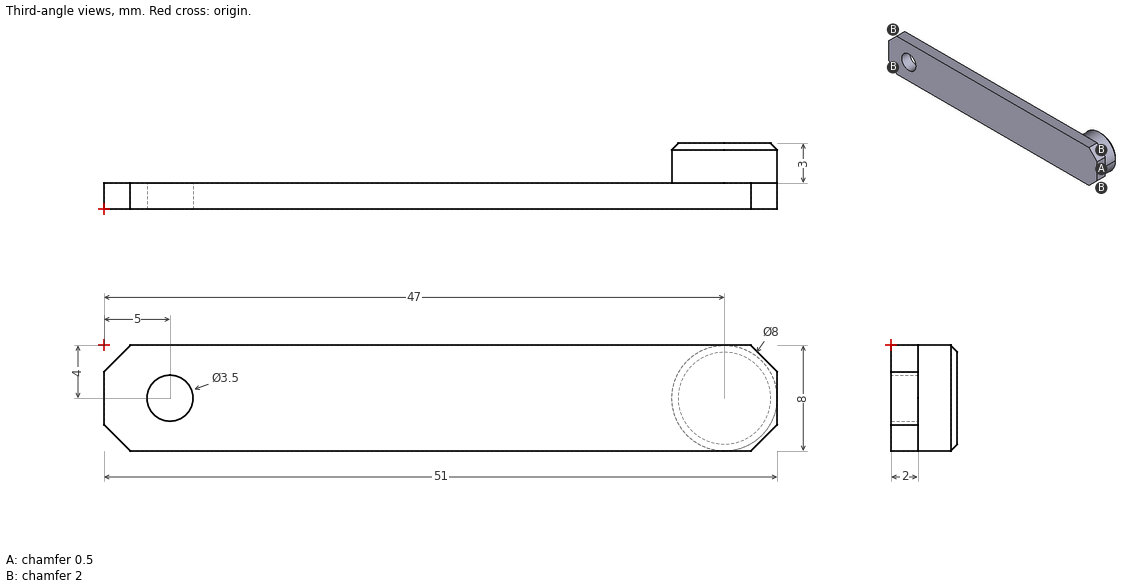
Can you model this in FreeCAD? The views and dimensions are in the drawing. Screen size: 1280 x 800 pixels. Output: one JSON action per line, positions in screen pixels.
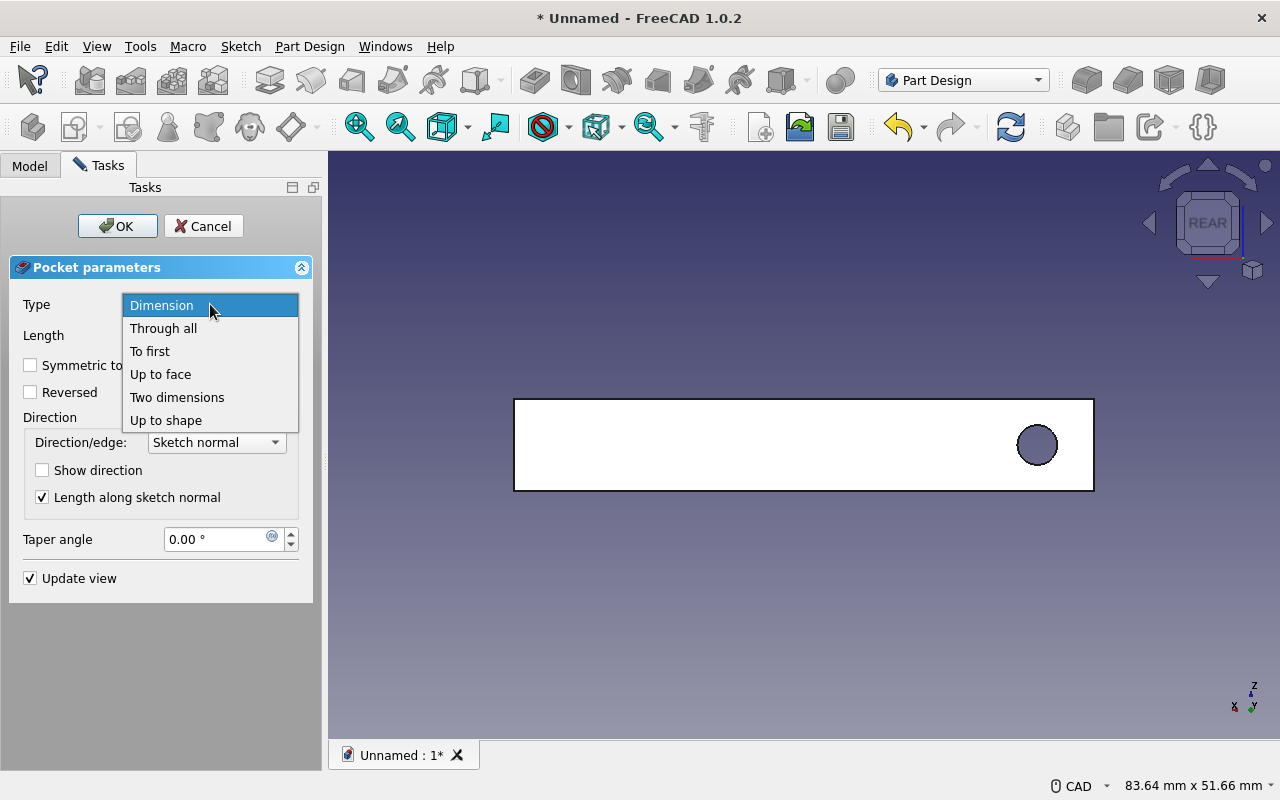
{"action": "left_click", "coordinate": [208, 328]}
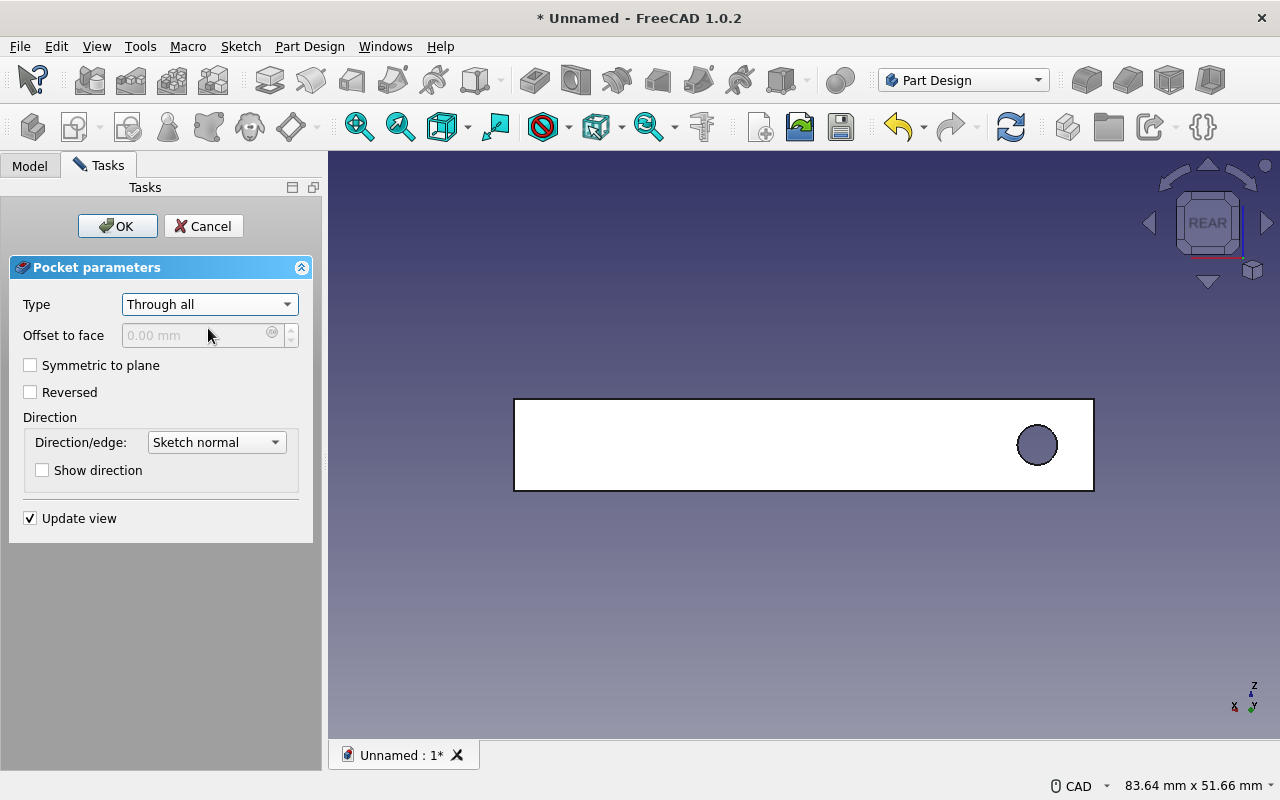
{"action": "left_click", "coordinate": [118, 226]}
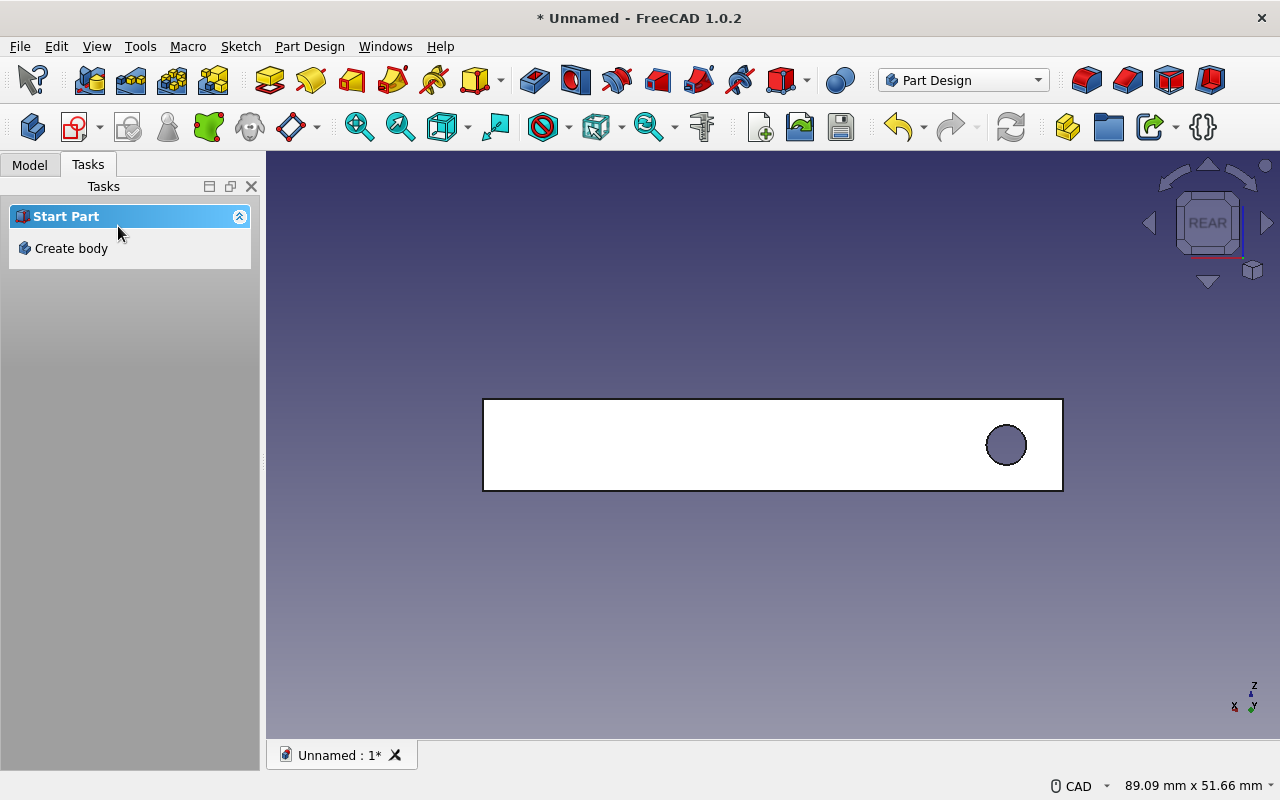
{"action": "left_click", "coordinate": [607, 444]}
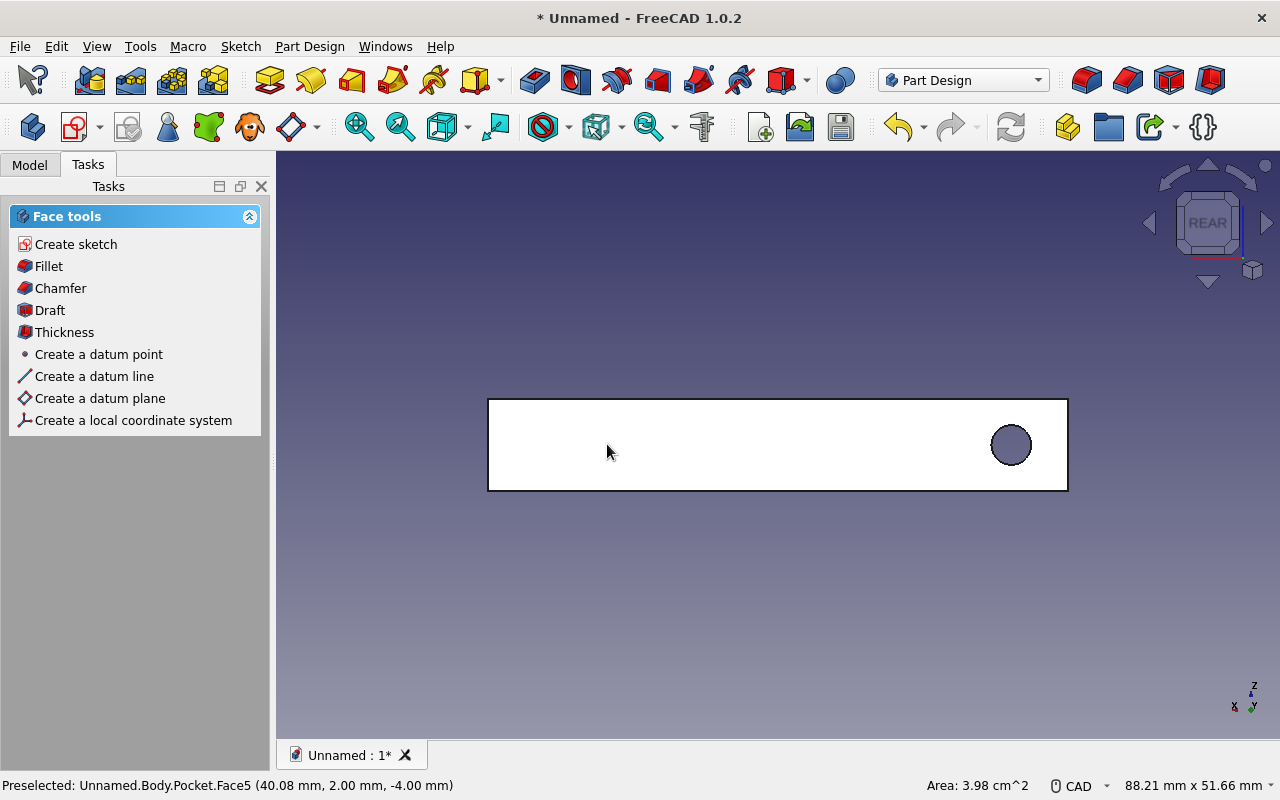
{"action": "left_click", "coordinate": [74, 128]}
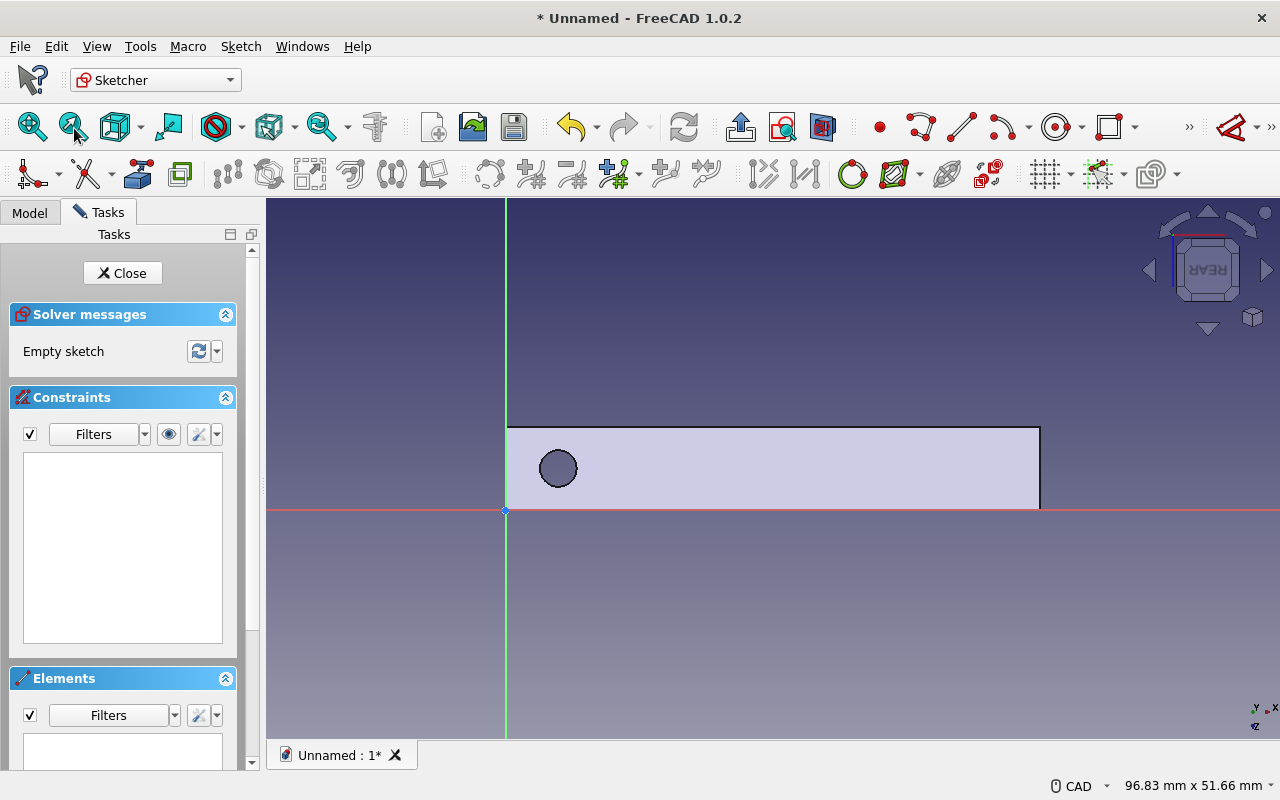
{"action": "scroll", "coordinate": [1094, 468], "scroll_direction": "up", "scroll_amount": 7}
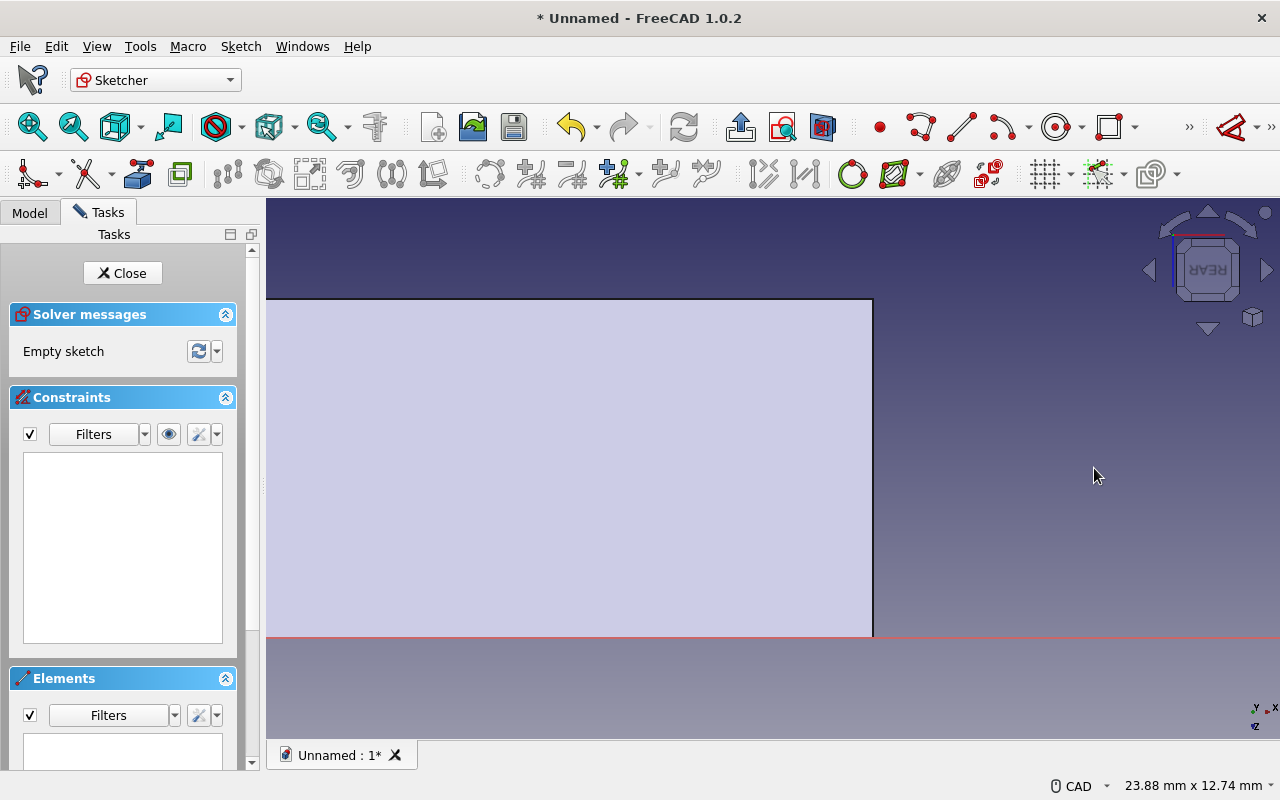
{"action": "key", "text": "g c"}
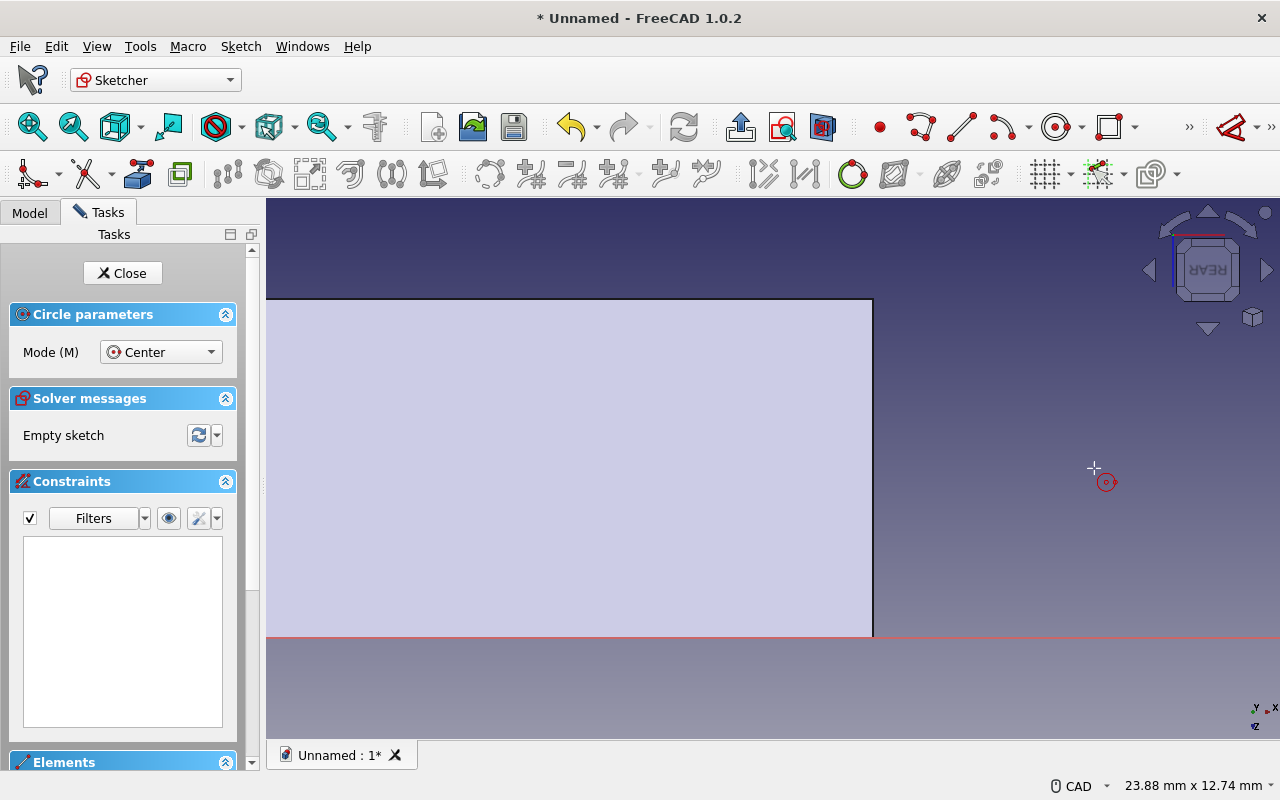
{"action": "left_click", "coordinate": [703, 468]}
{"action": "mouse_move", "coordinate": [823, 348]}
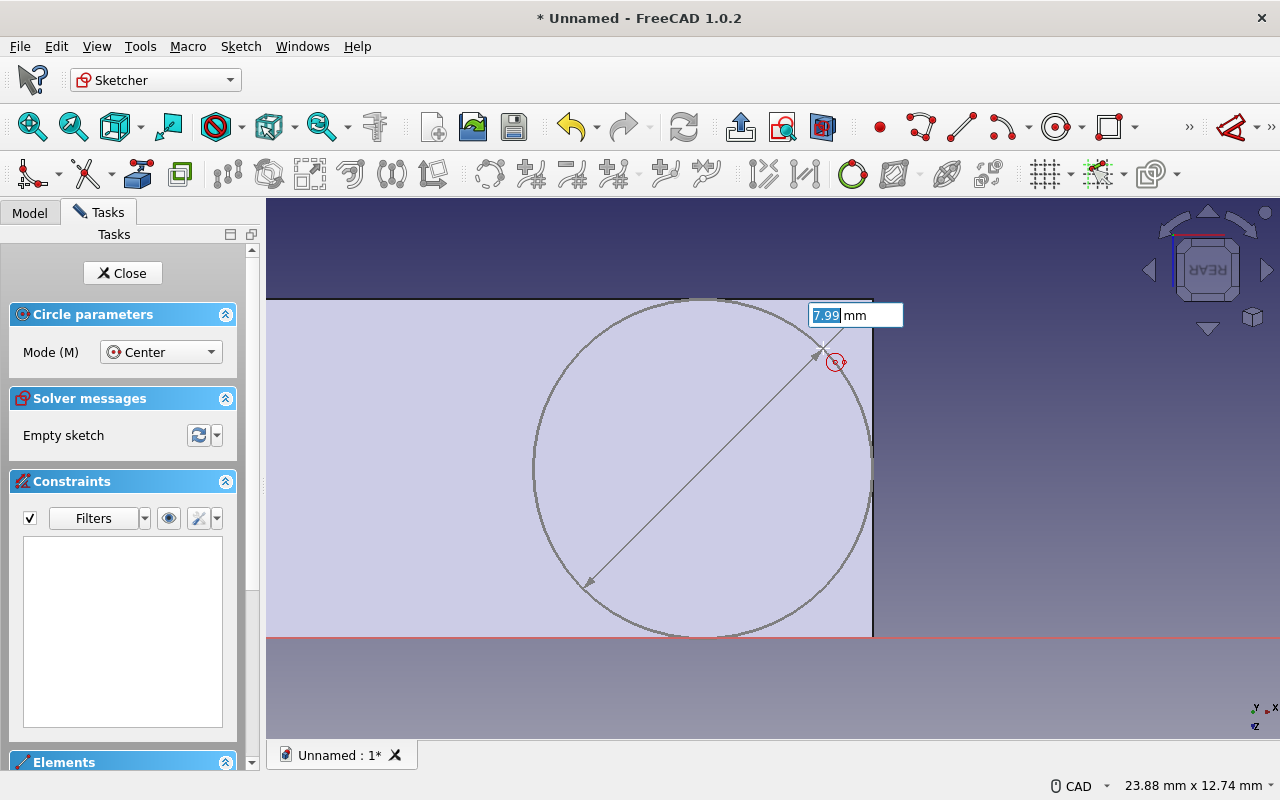
{"action": "type", "text": "8"}
{"action": "key", "text": "Return"}
{"action": "key", "text": "Escape"}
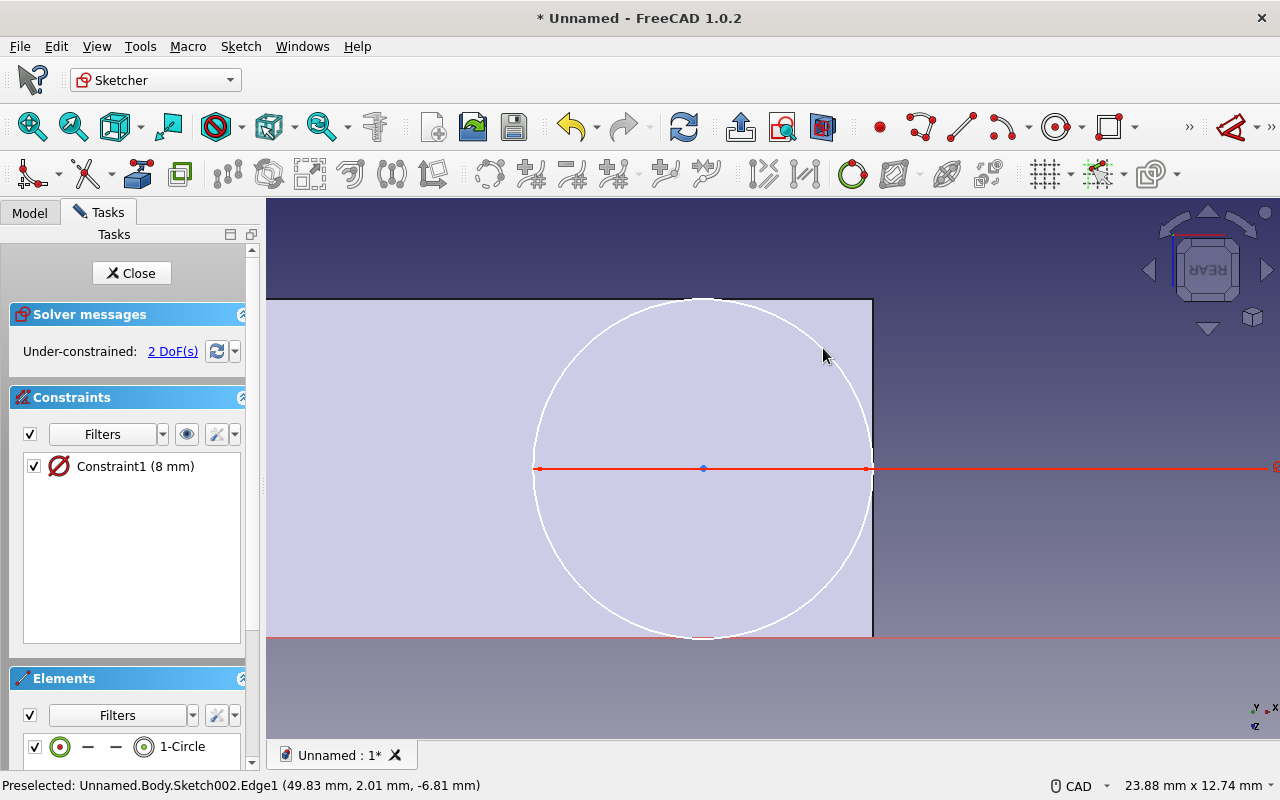
{"action": "left_click", "coordinate": [703, 469]}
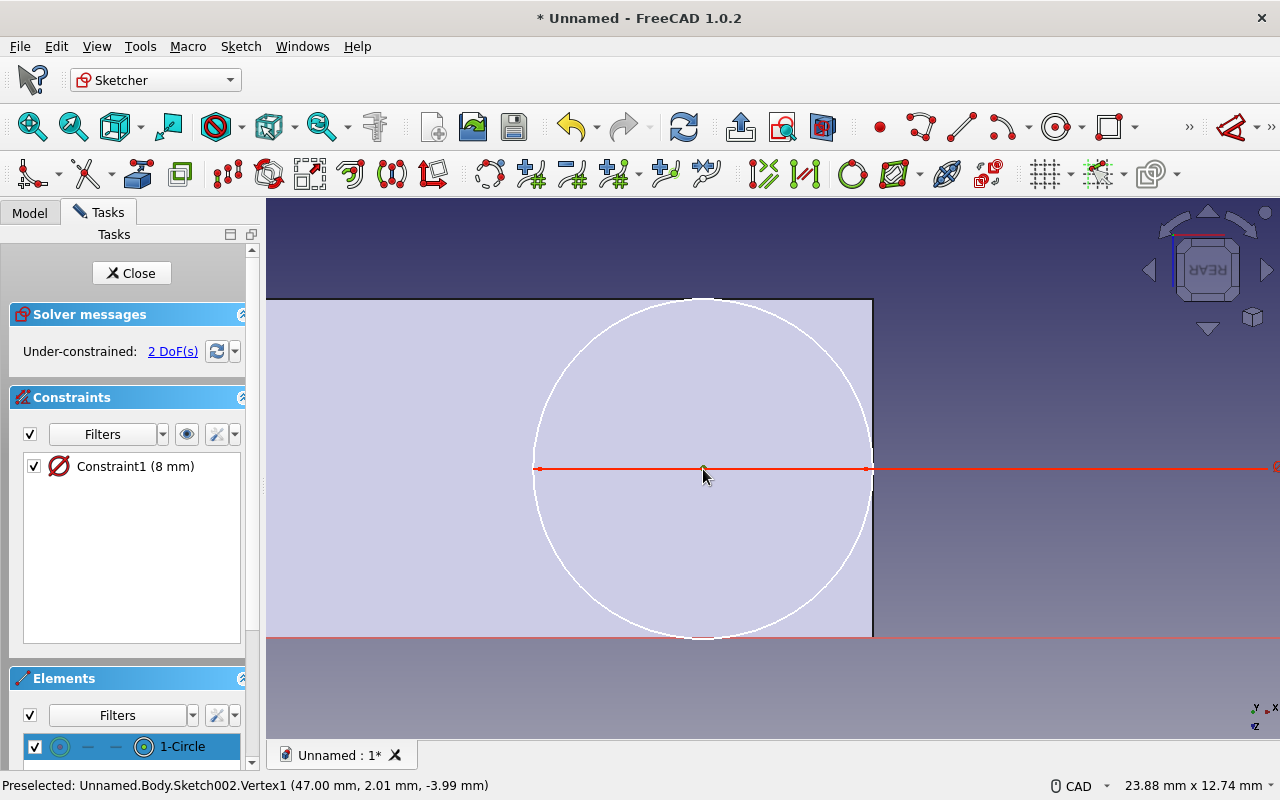
{"action": "key", "text": "i"}